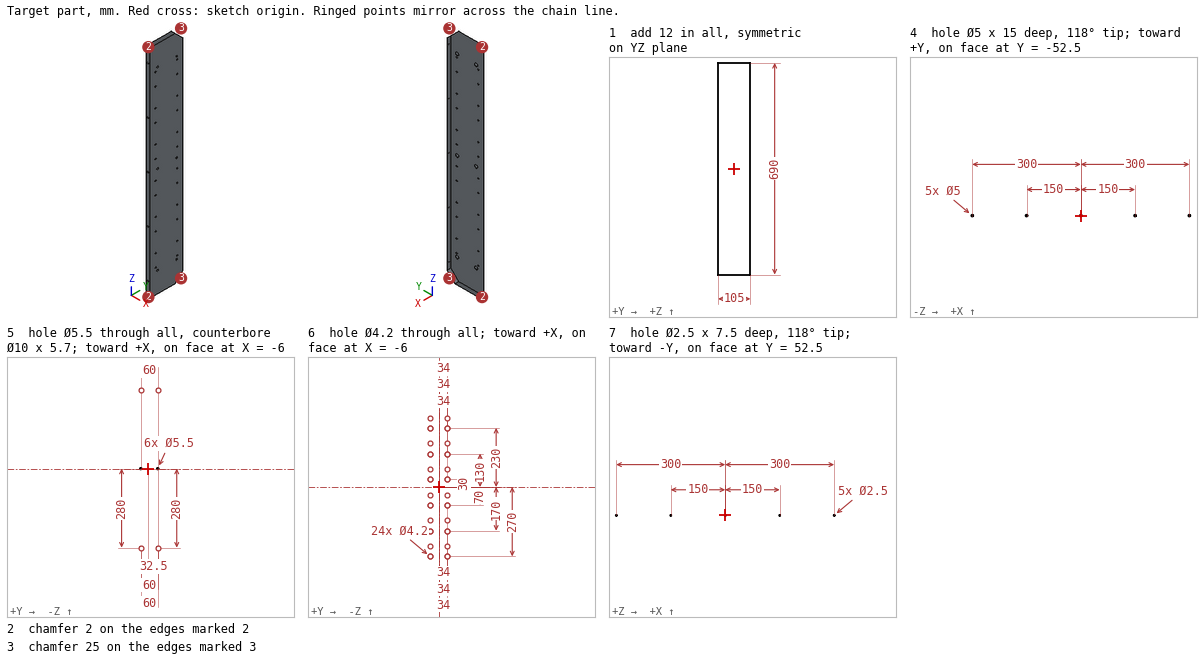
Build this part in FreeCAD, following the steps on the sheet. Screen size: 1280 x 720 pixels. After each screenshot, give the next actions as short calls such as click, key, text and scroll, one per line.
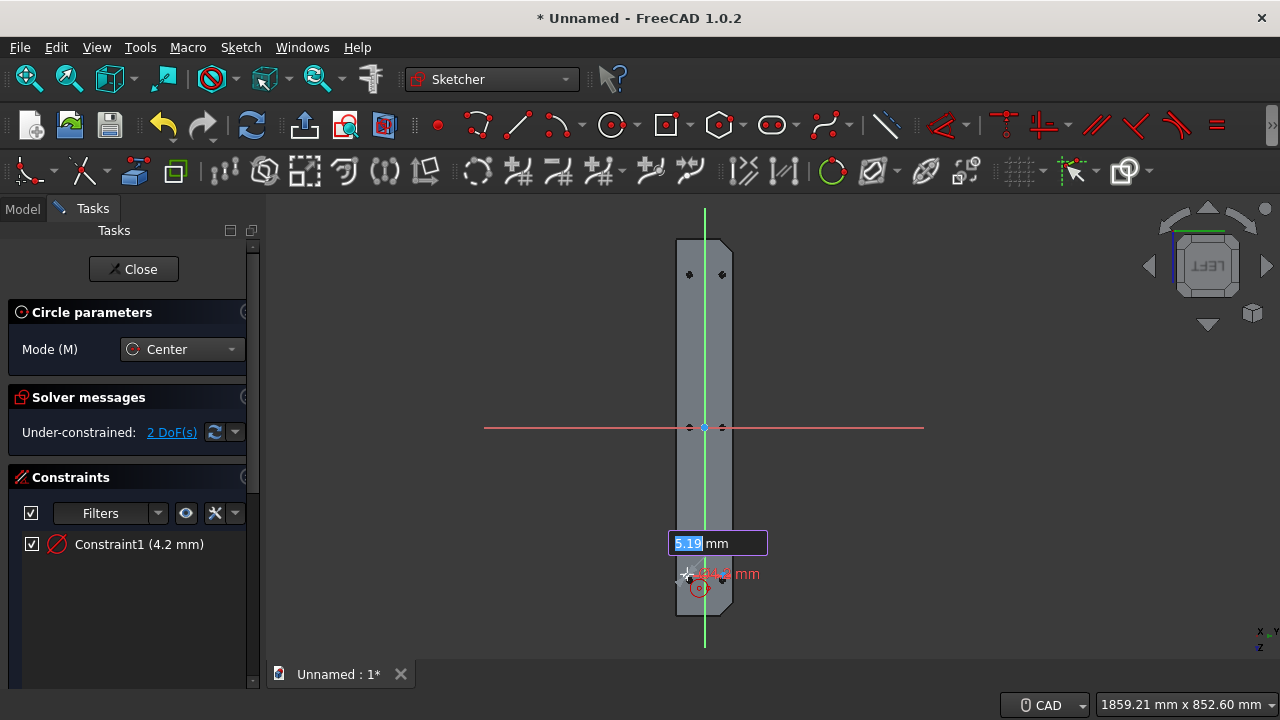
text(4.2)
key(Return)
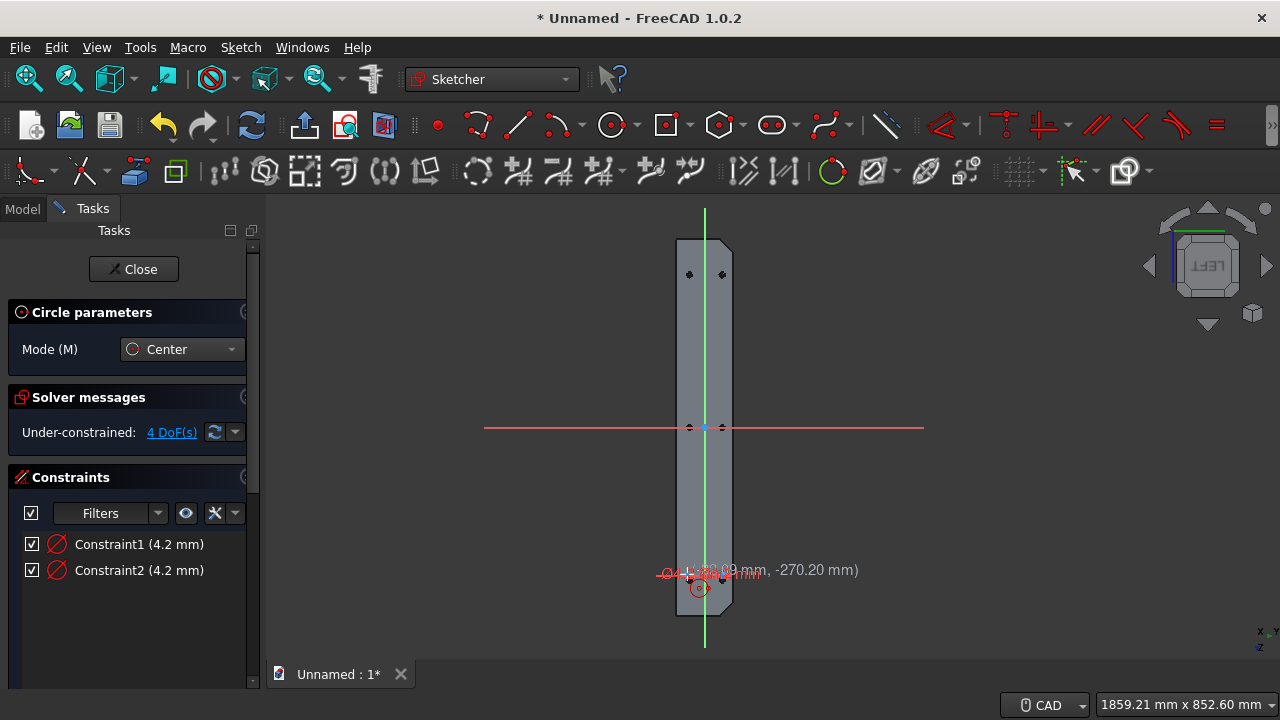
scroll(723, 520, up, 15)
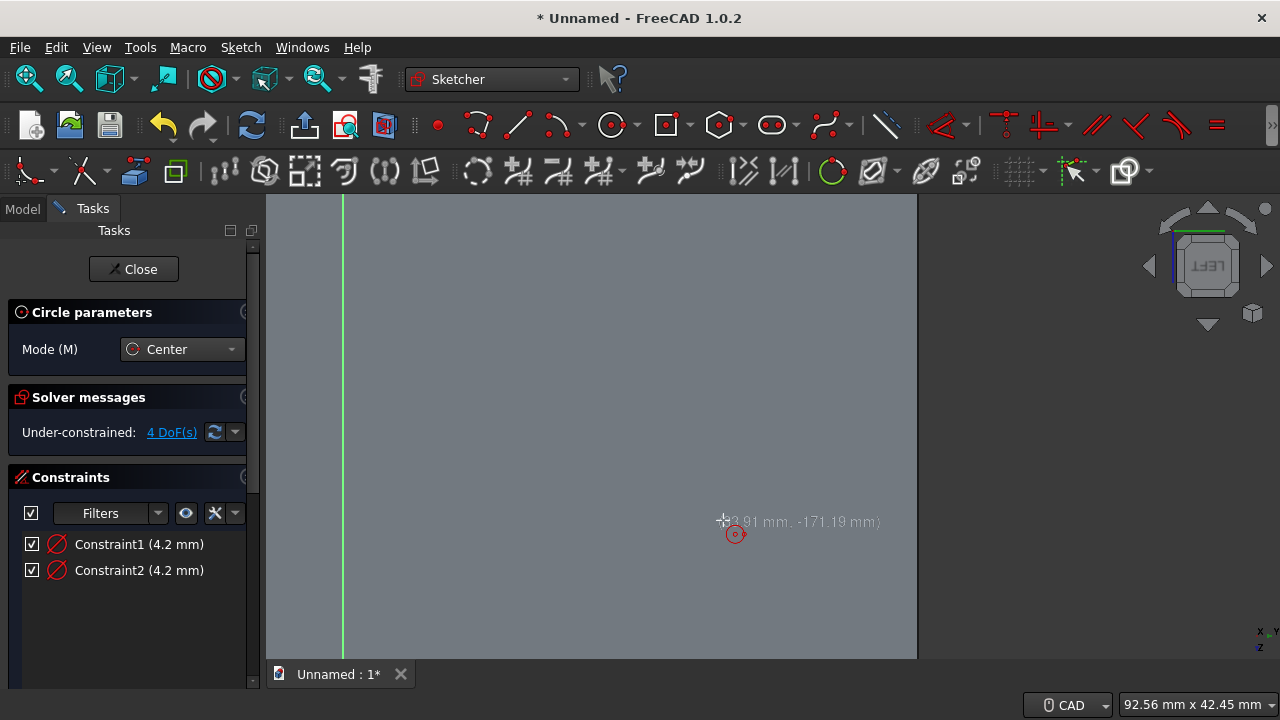
scroll(723, 520, down, 15)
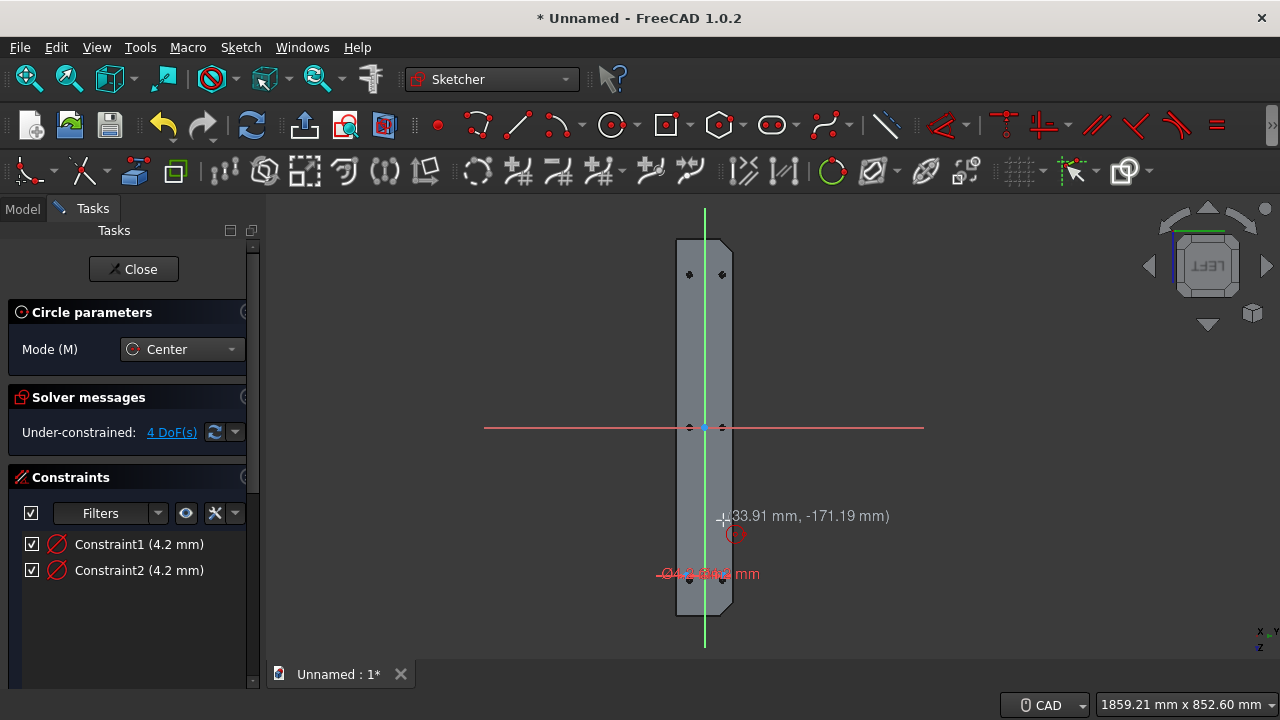
click(723, 520)
move(724, 520)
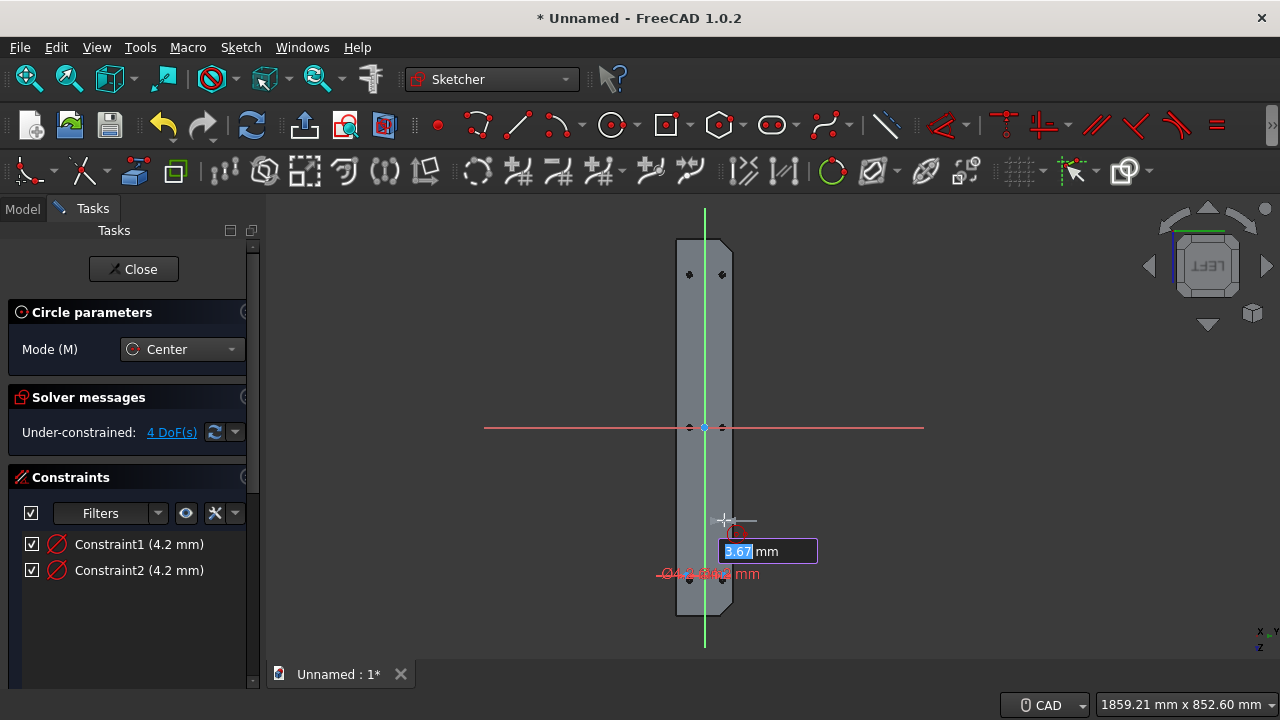
text(4.2)
key(Return)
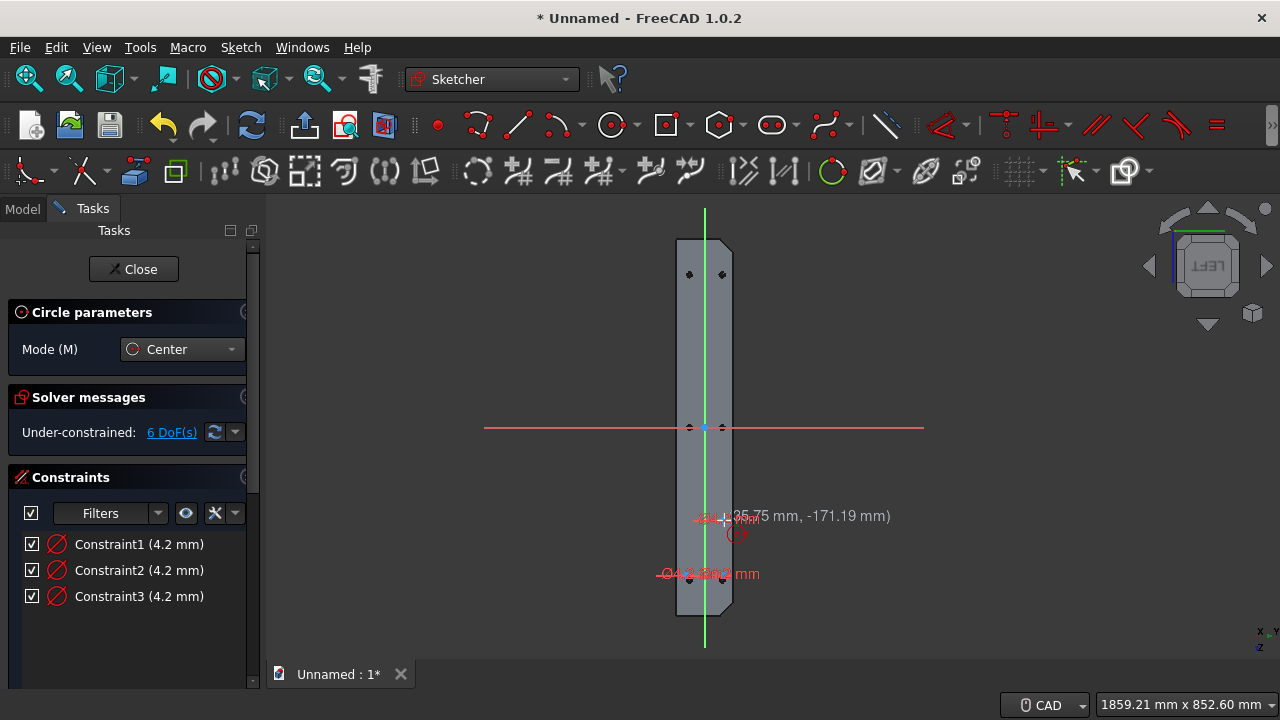
scroll(686, 520, up, 15)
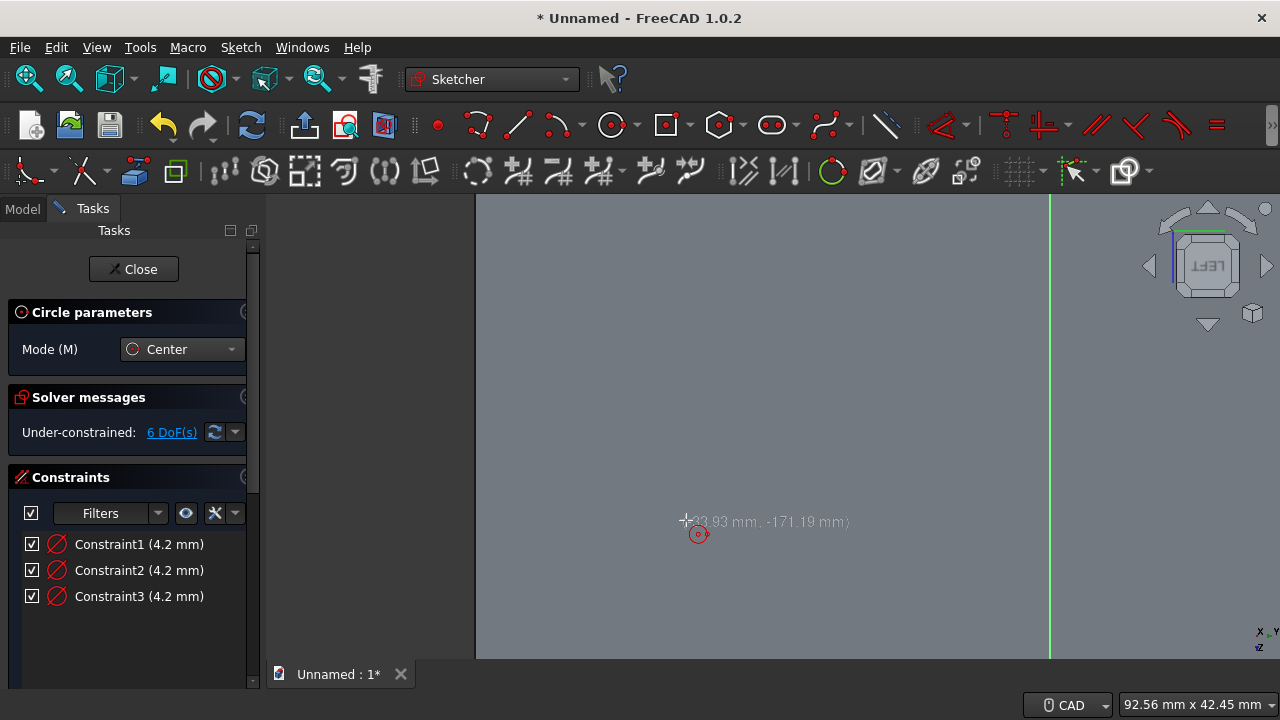
scroll(686, 520, down, 15)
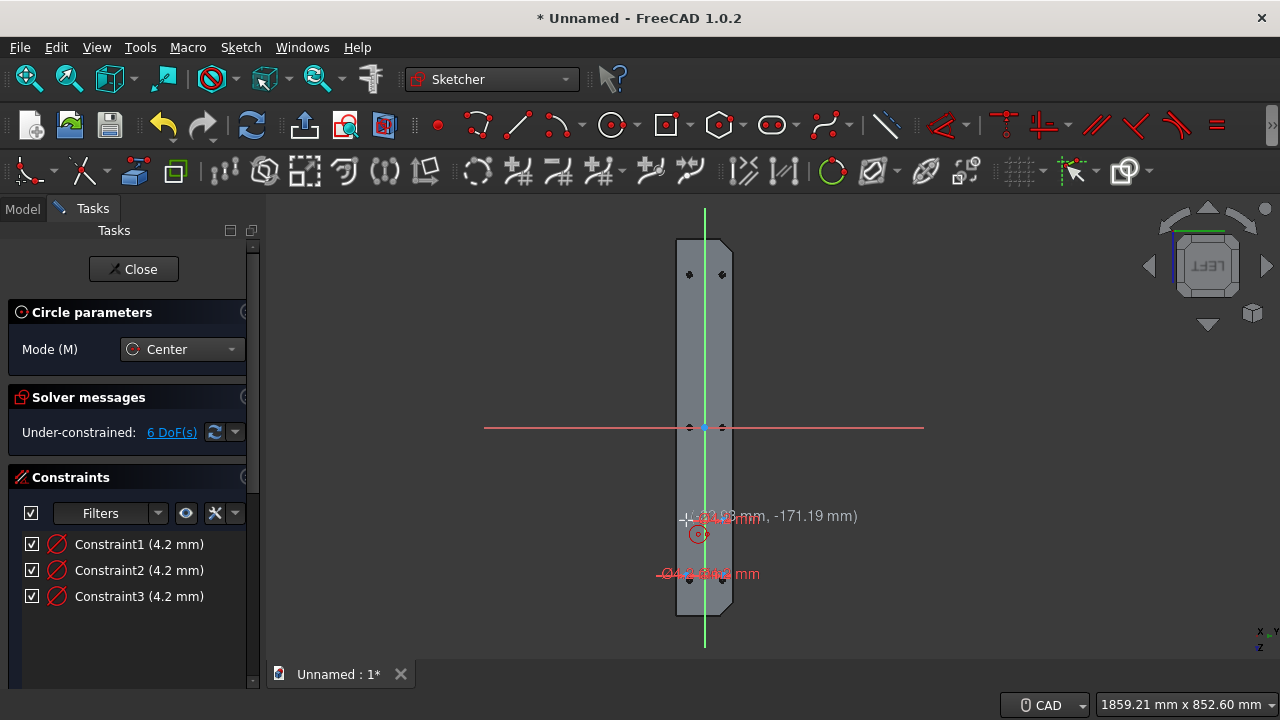
click(686, 520)
move(687, 520)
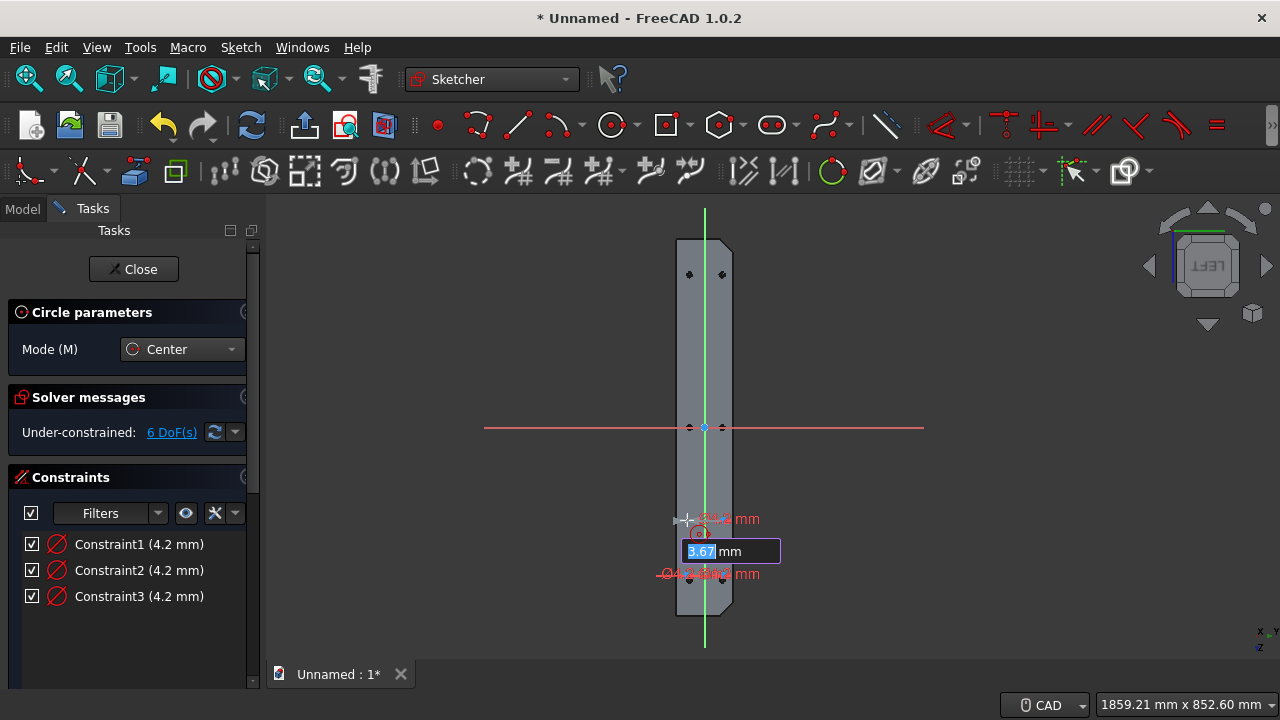
text(4.2)
key(Return)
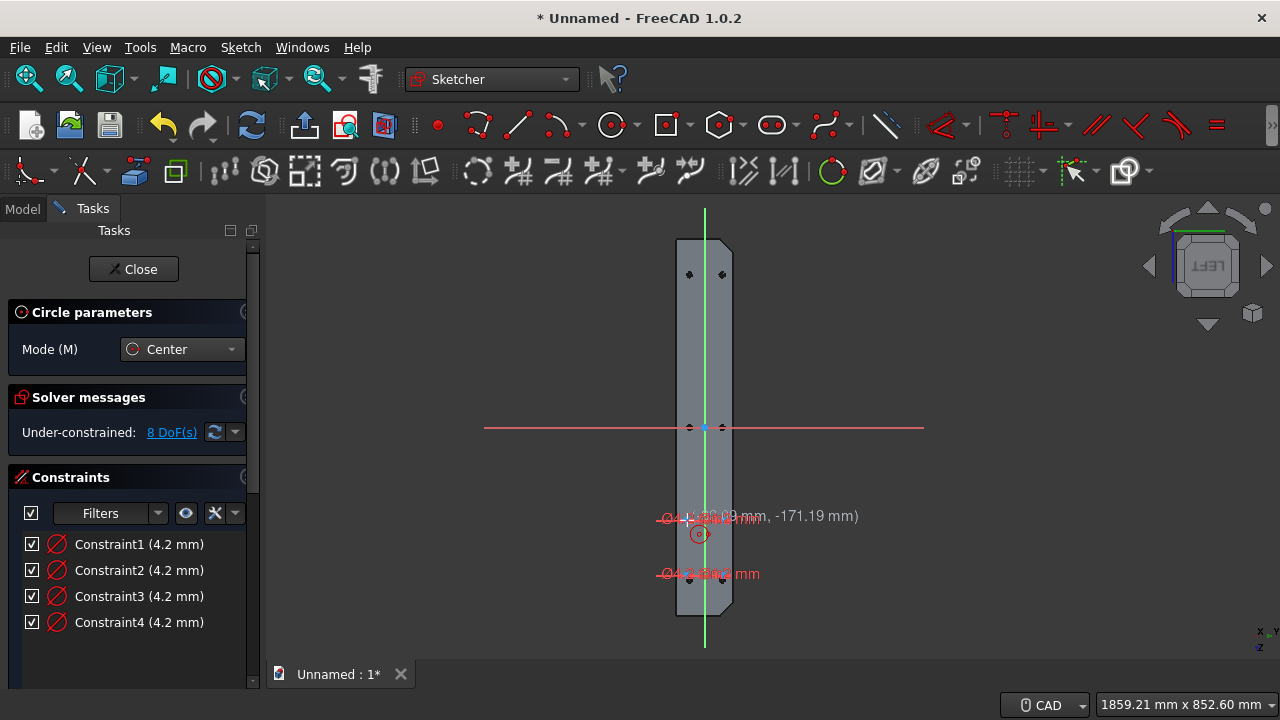
scroll(723, 466, up, 15)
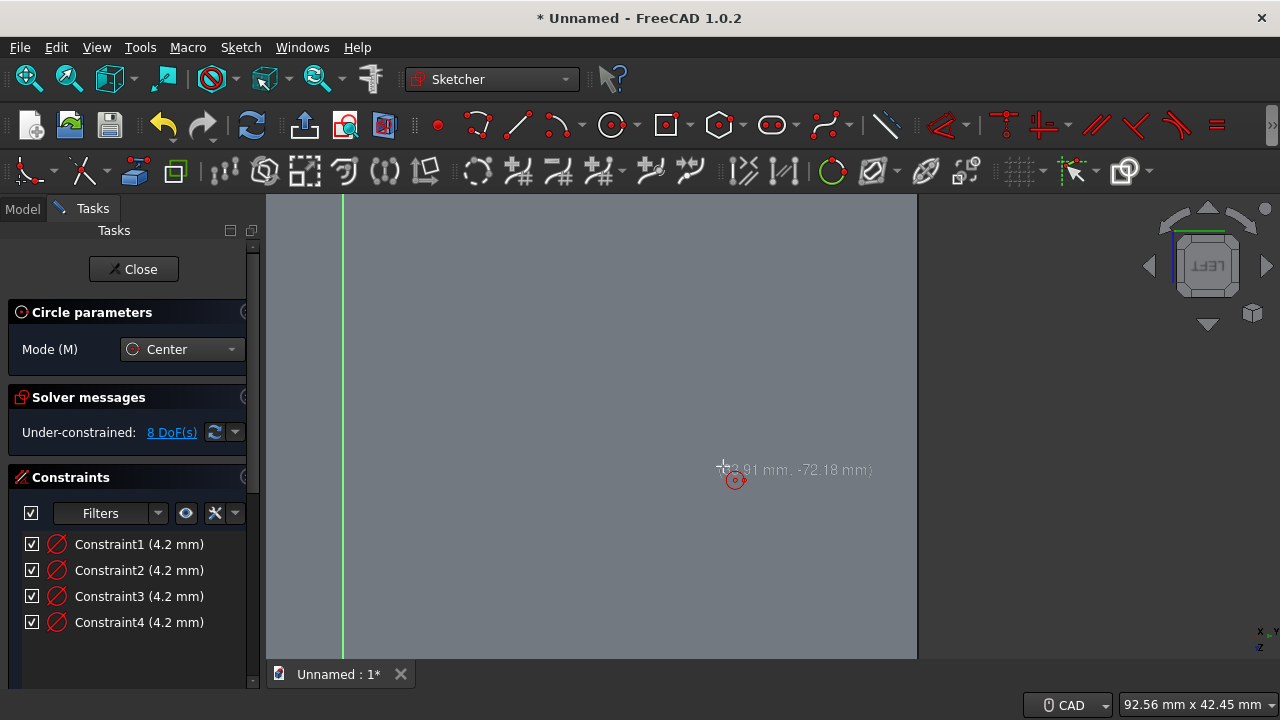
scroll(723, 465, down, 15)